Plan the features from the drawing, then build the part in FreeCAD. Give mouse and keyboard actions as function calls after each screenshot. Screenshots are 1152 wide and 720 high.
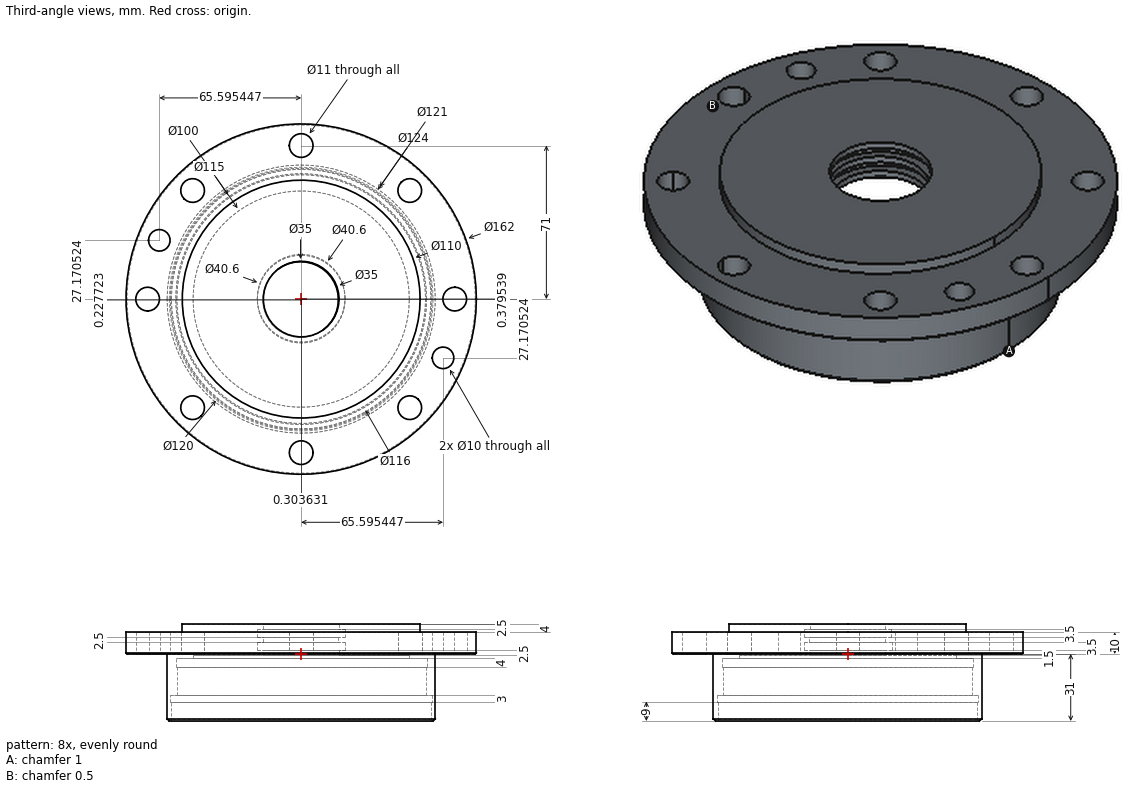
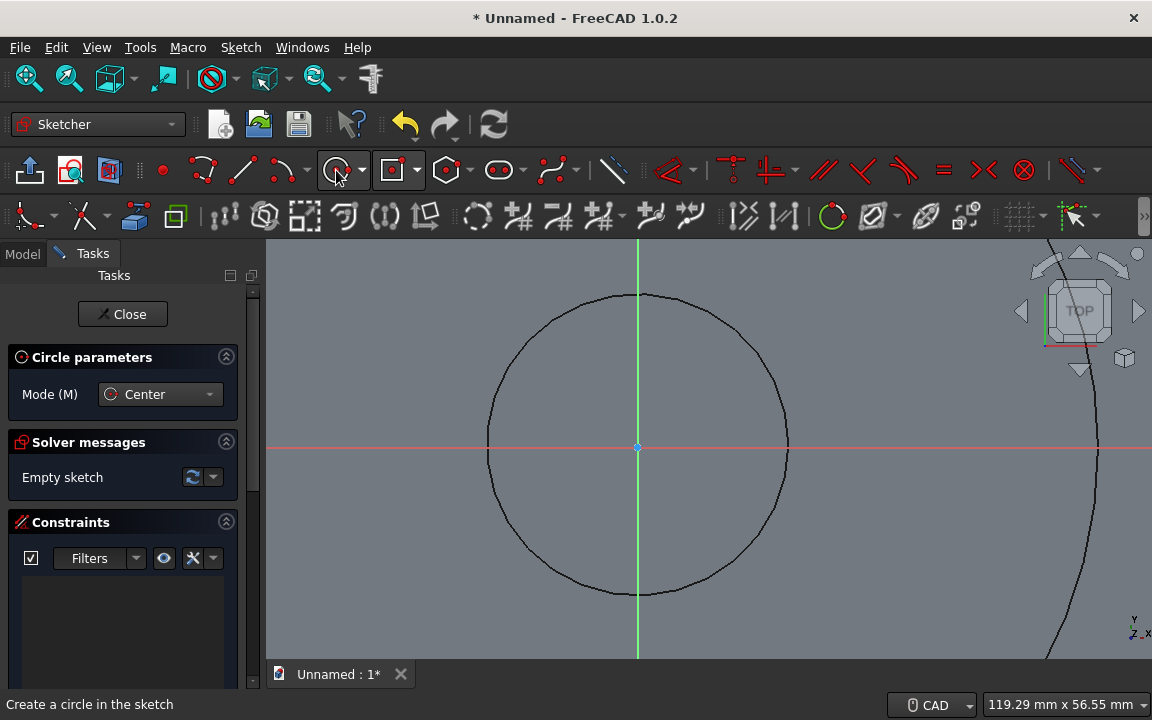
click(638, 448)
click(729, 356)
key(Escape)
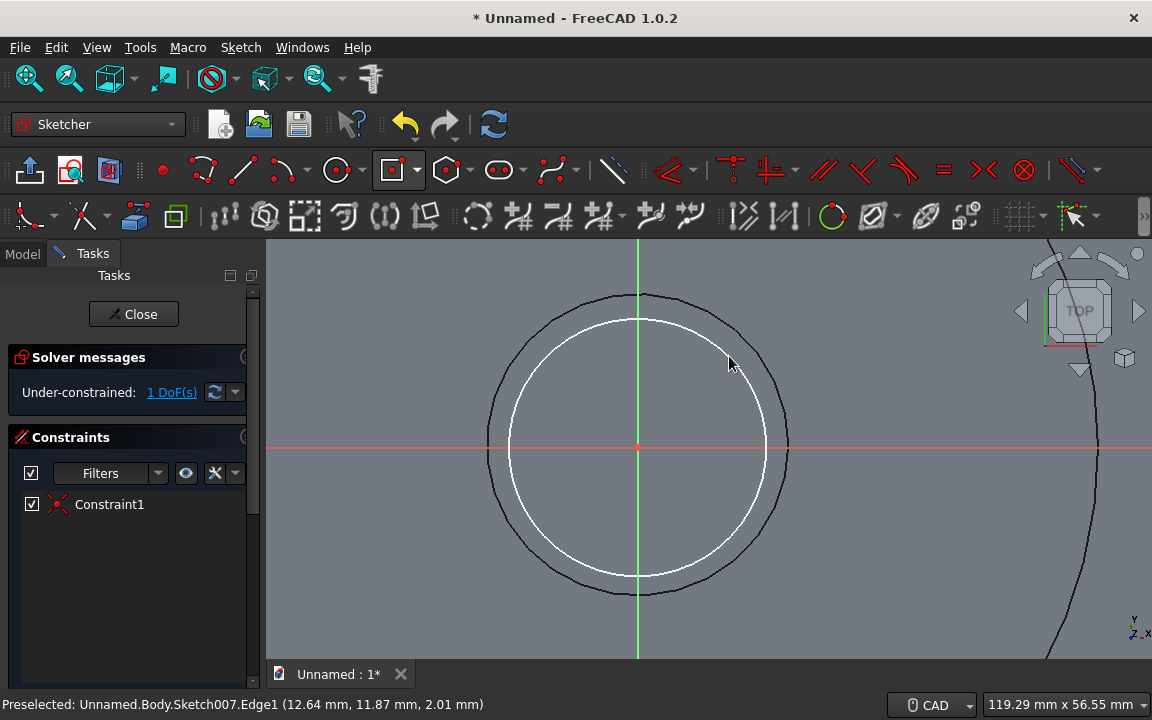
click(668, 170)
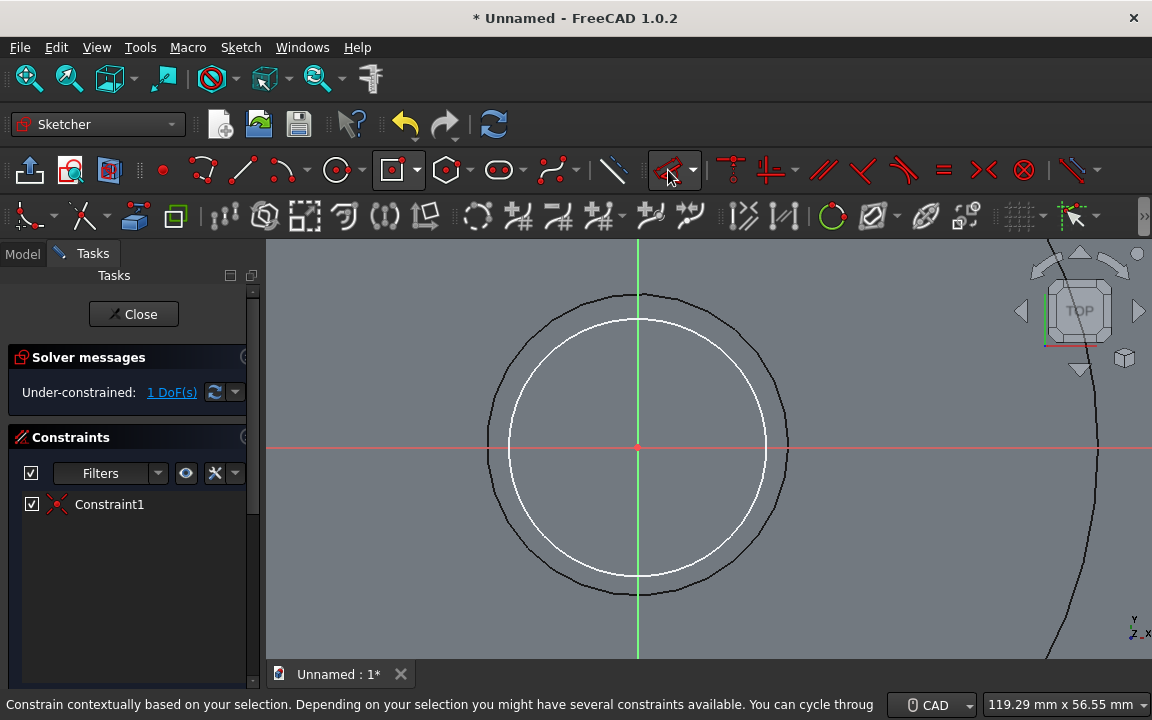
click(728, 356)
click(750, 333)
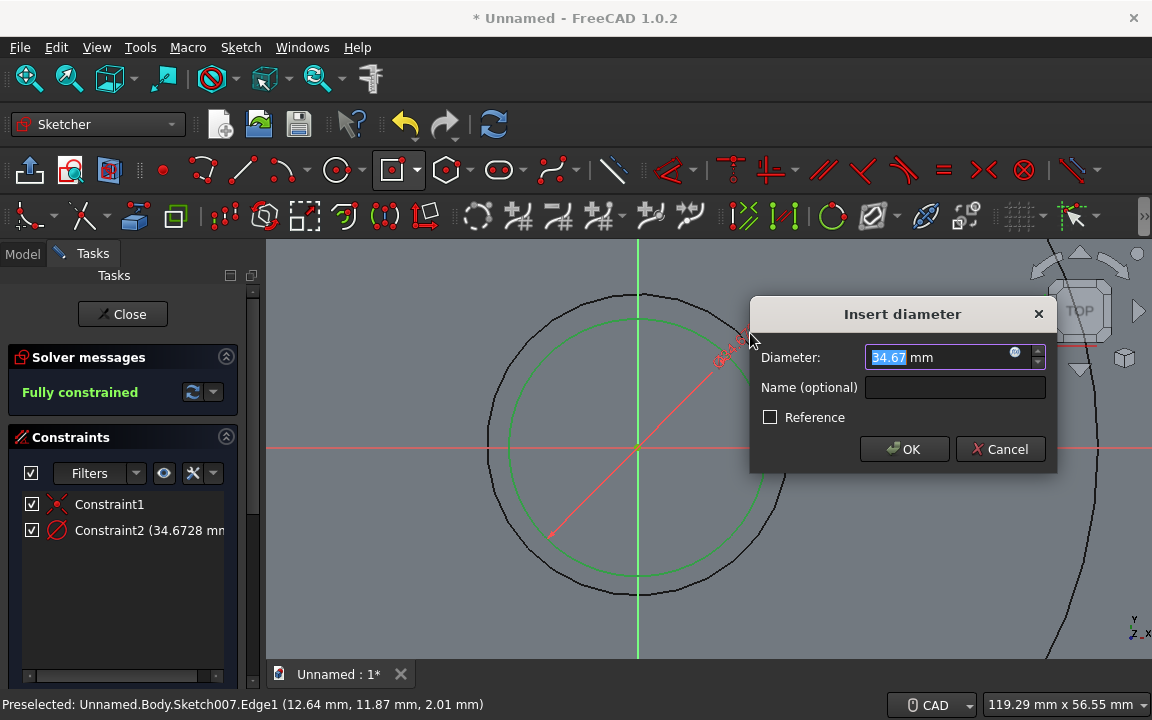
text(35)
key(Return)
key(Escape)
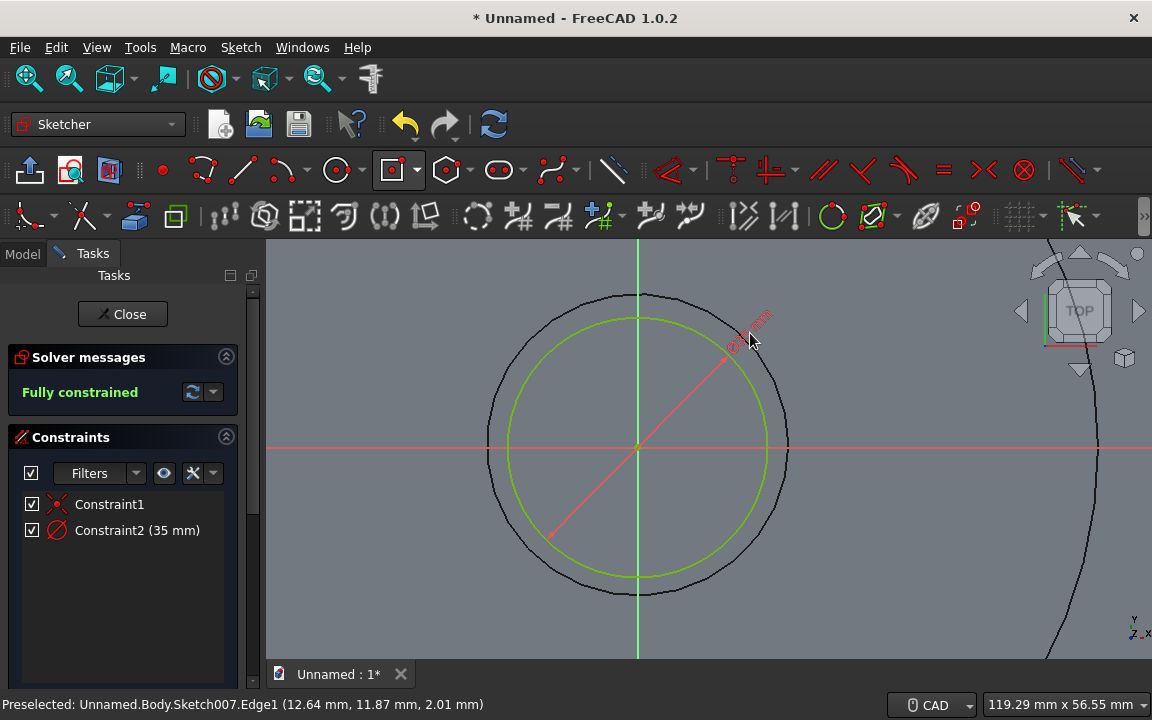
click(123, 314)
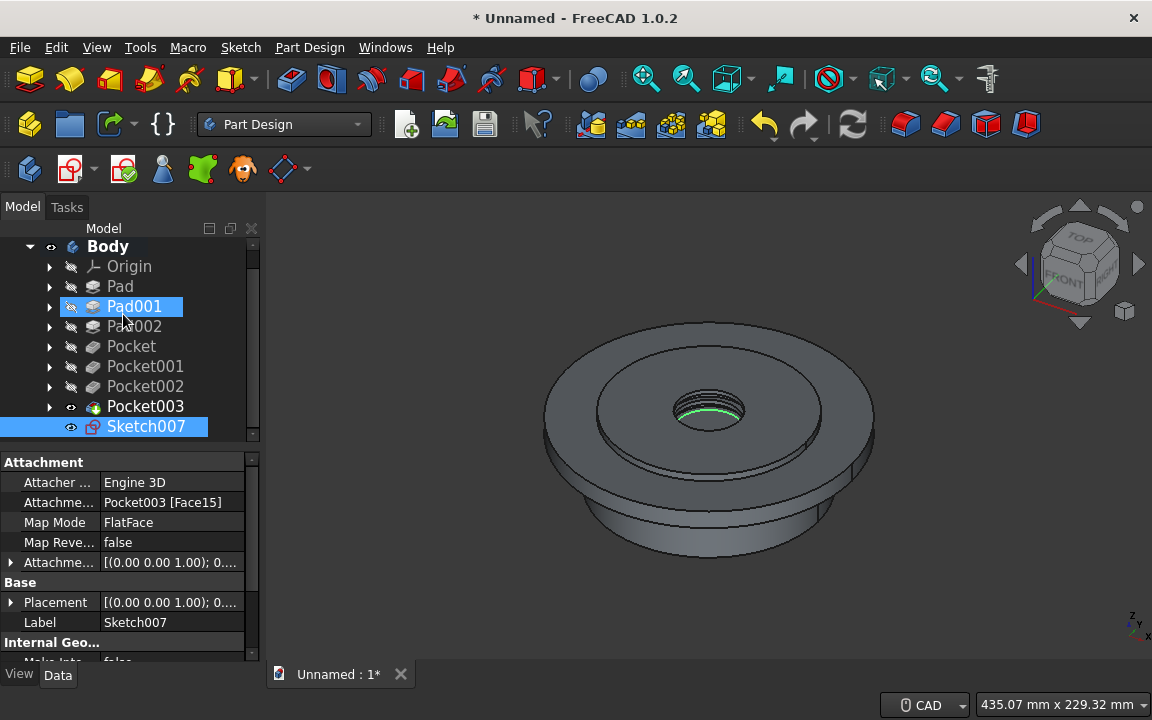
click(292, 80)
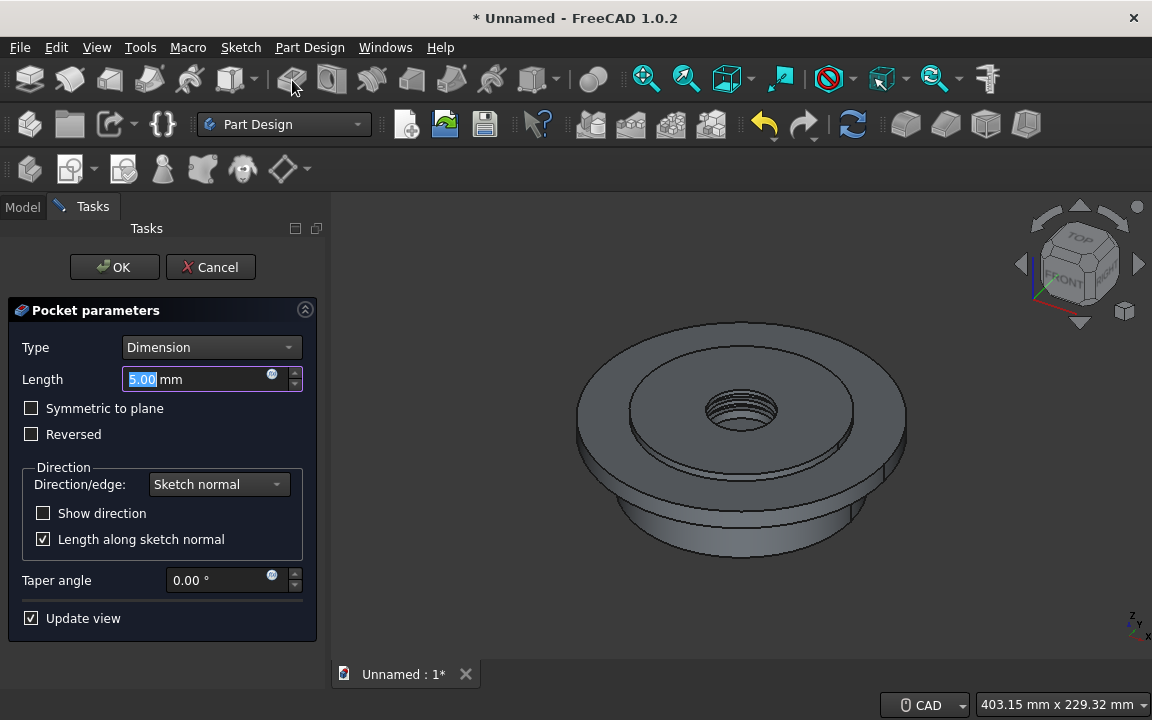
text(2.5)
key(Tab)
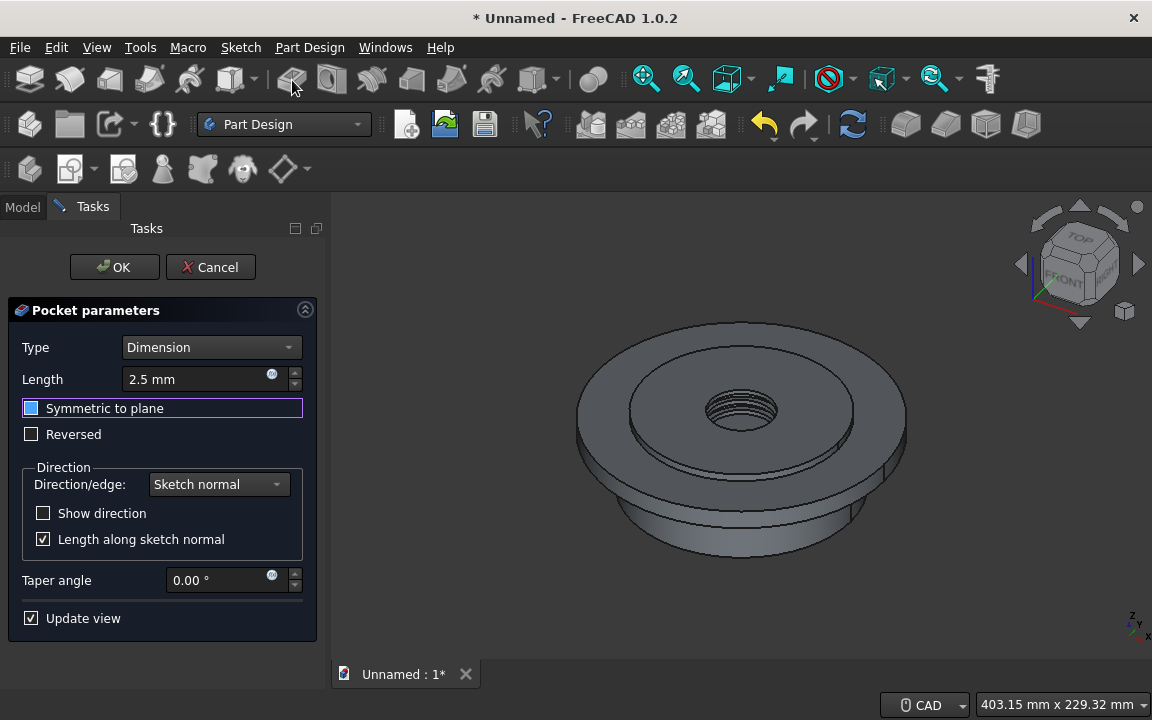
click(115, 267)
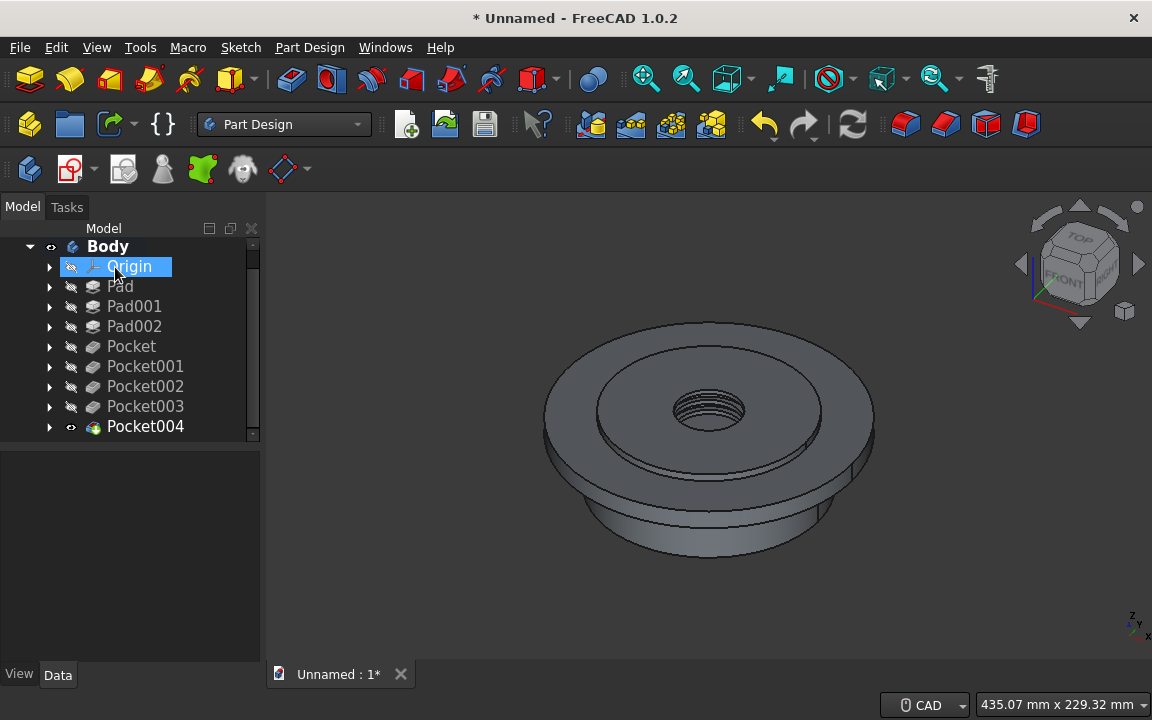
key(0)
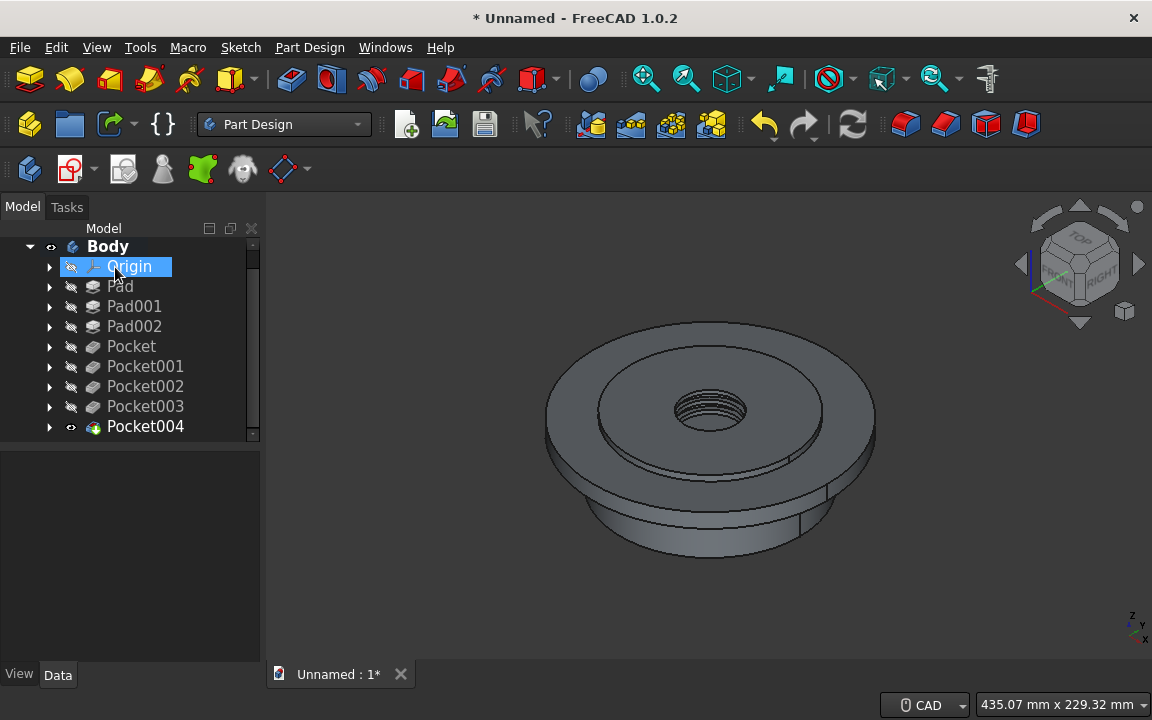
key(2)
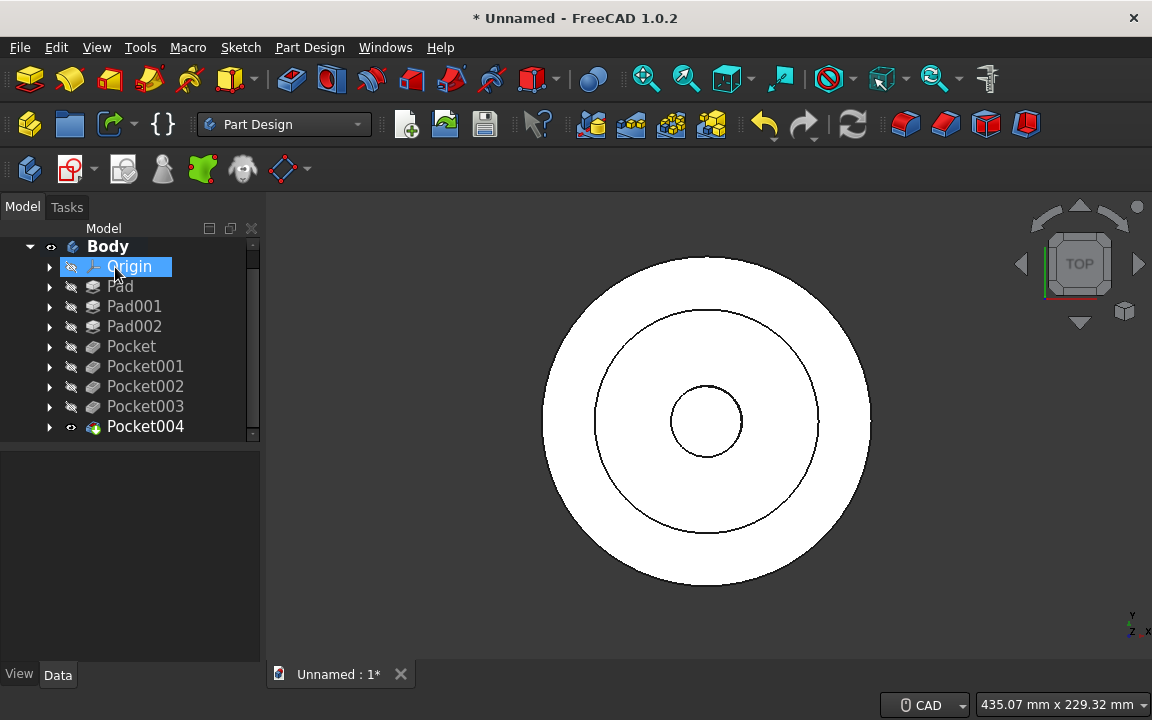
click(707, 420)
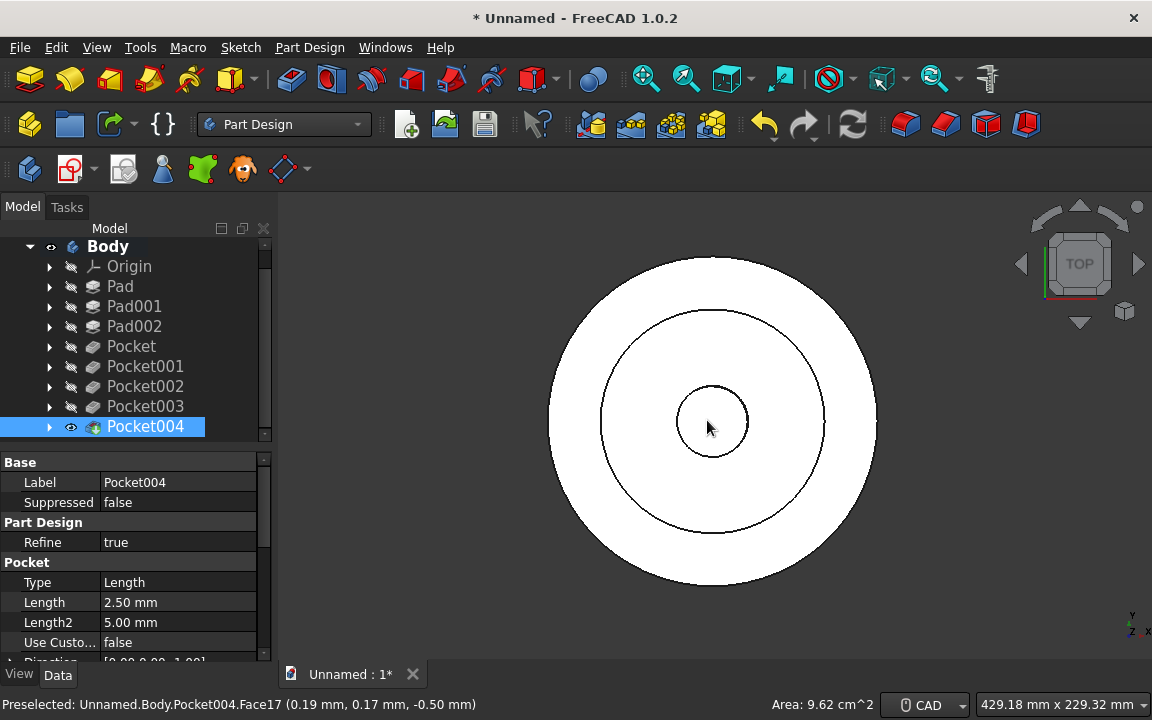
click(70, 170)